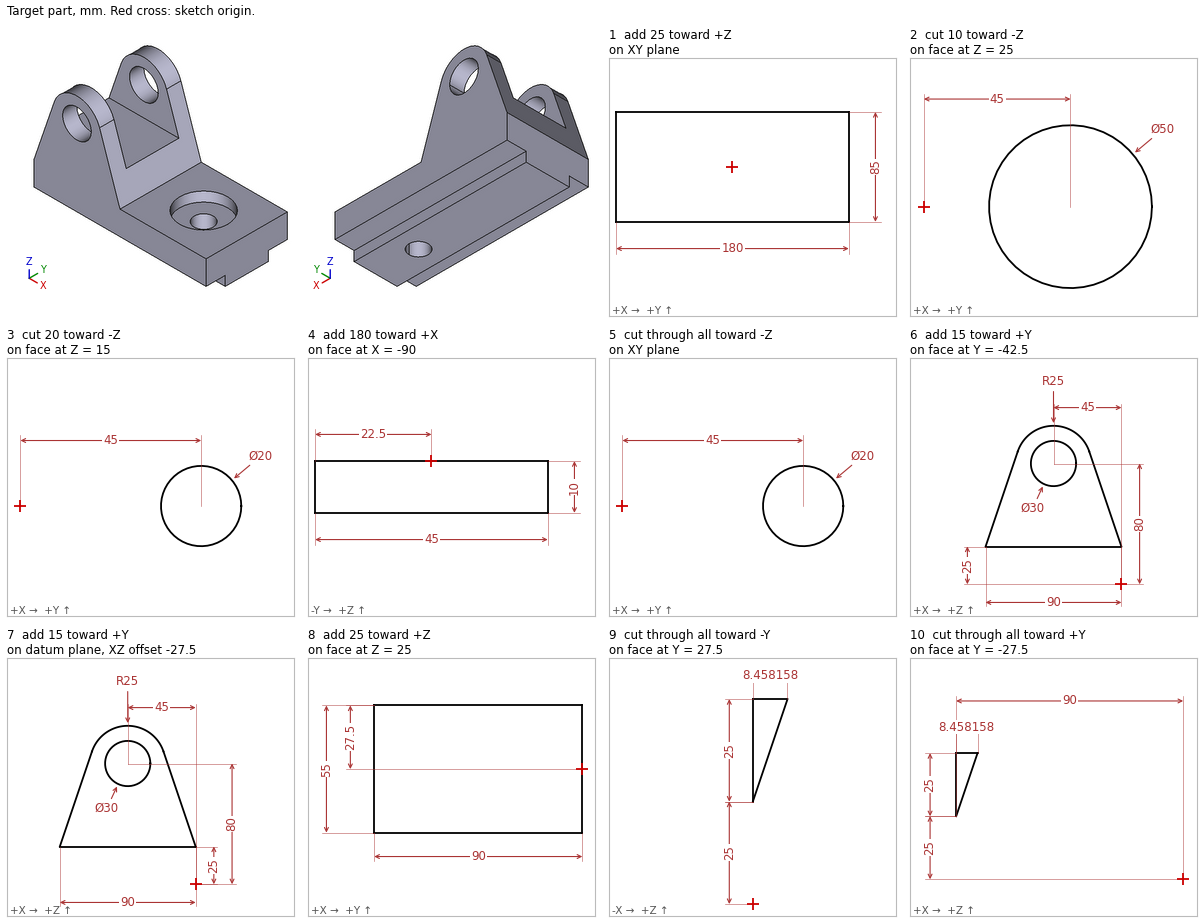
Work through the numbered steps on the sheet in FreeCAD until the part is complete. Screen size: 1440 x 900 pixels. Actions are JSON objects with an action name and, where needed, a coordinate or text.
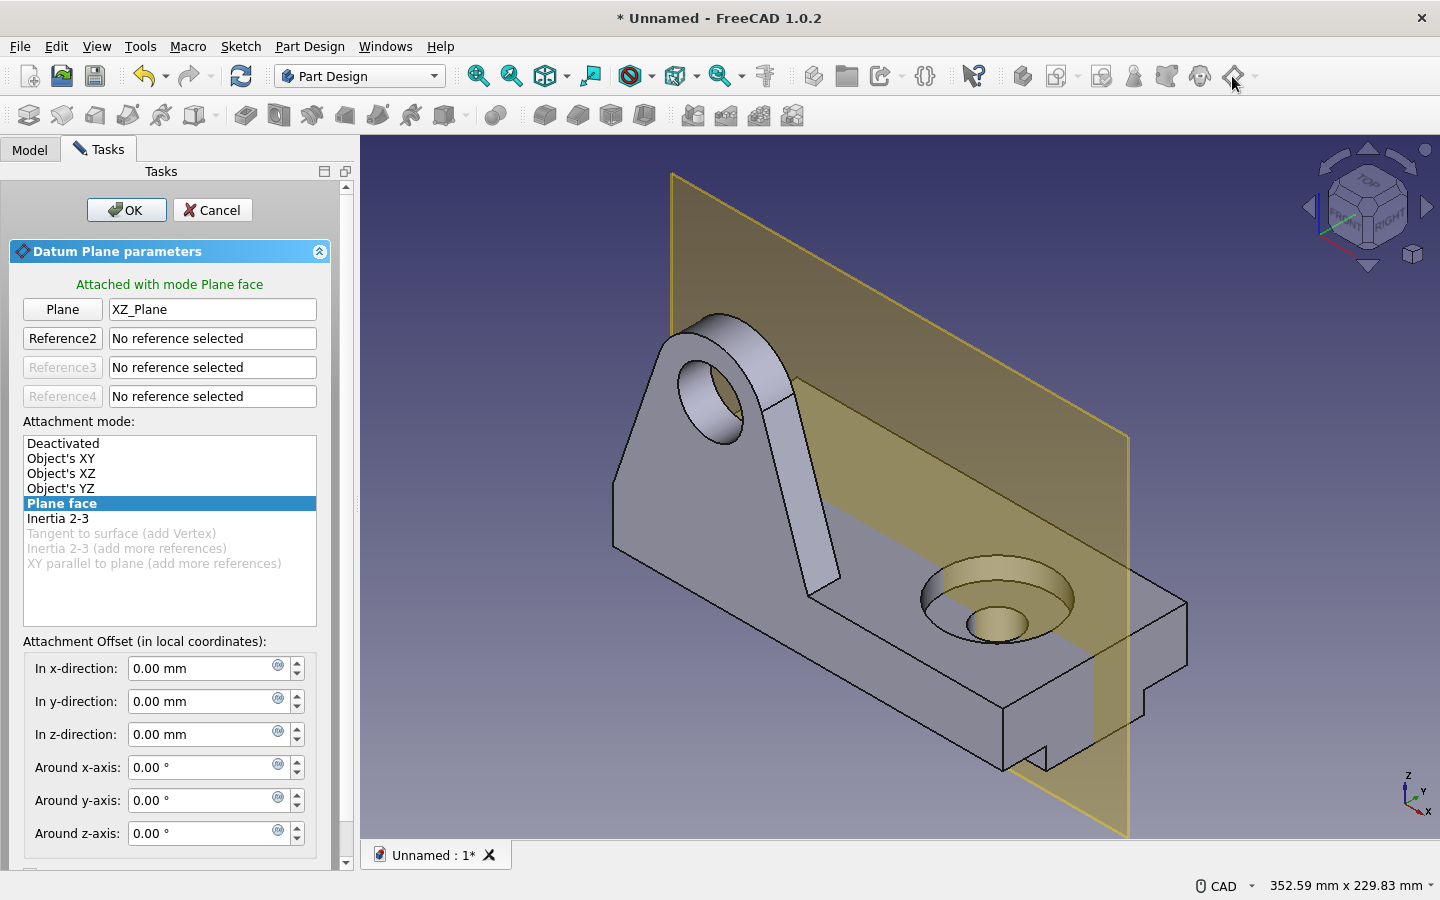
{"action": "triple_click", "coordinate": [210, 734]}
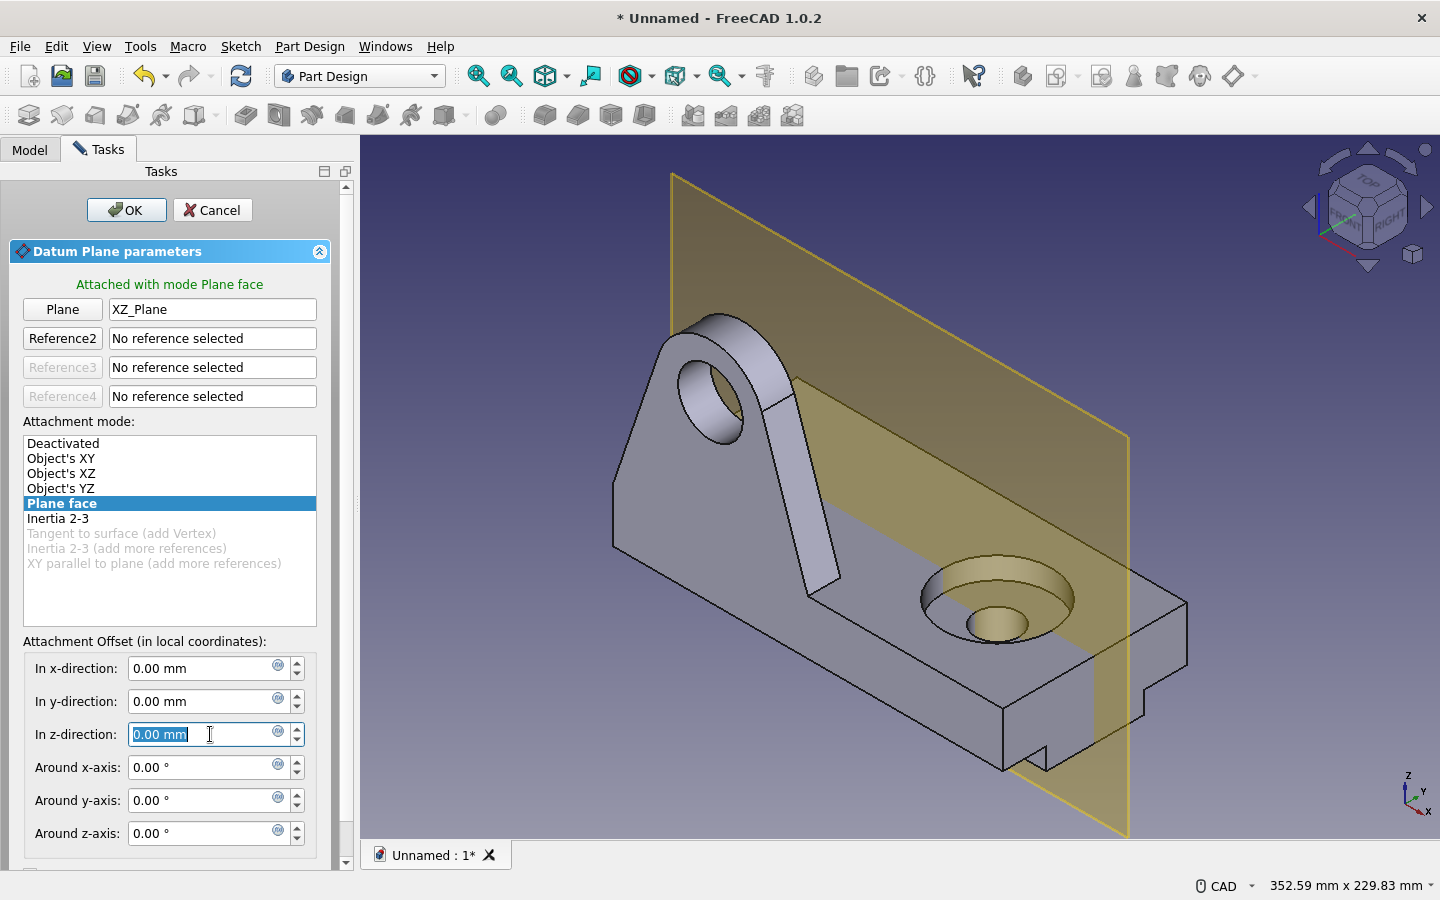
{"action": "type", "text": "-27.5"}
{"action": "key", "text": "Tab"}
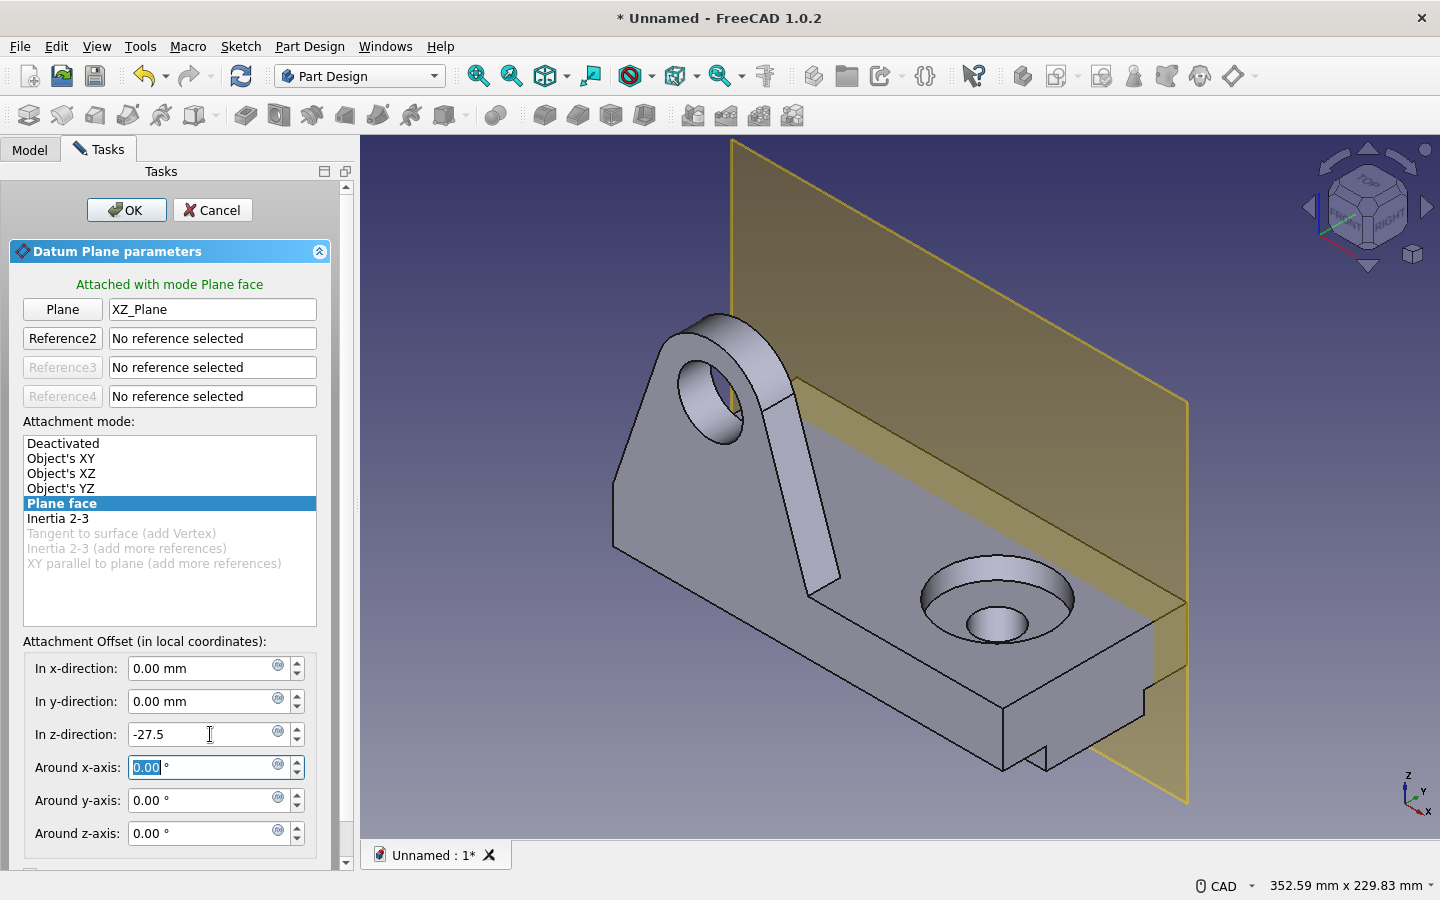
{"action": "left_click", "coordinate": [127, 210]}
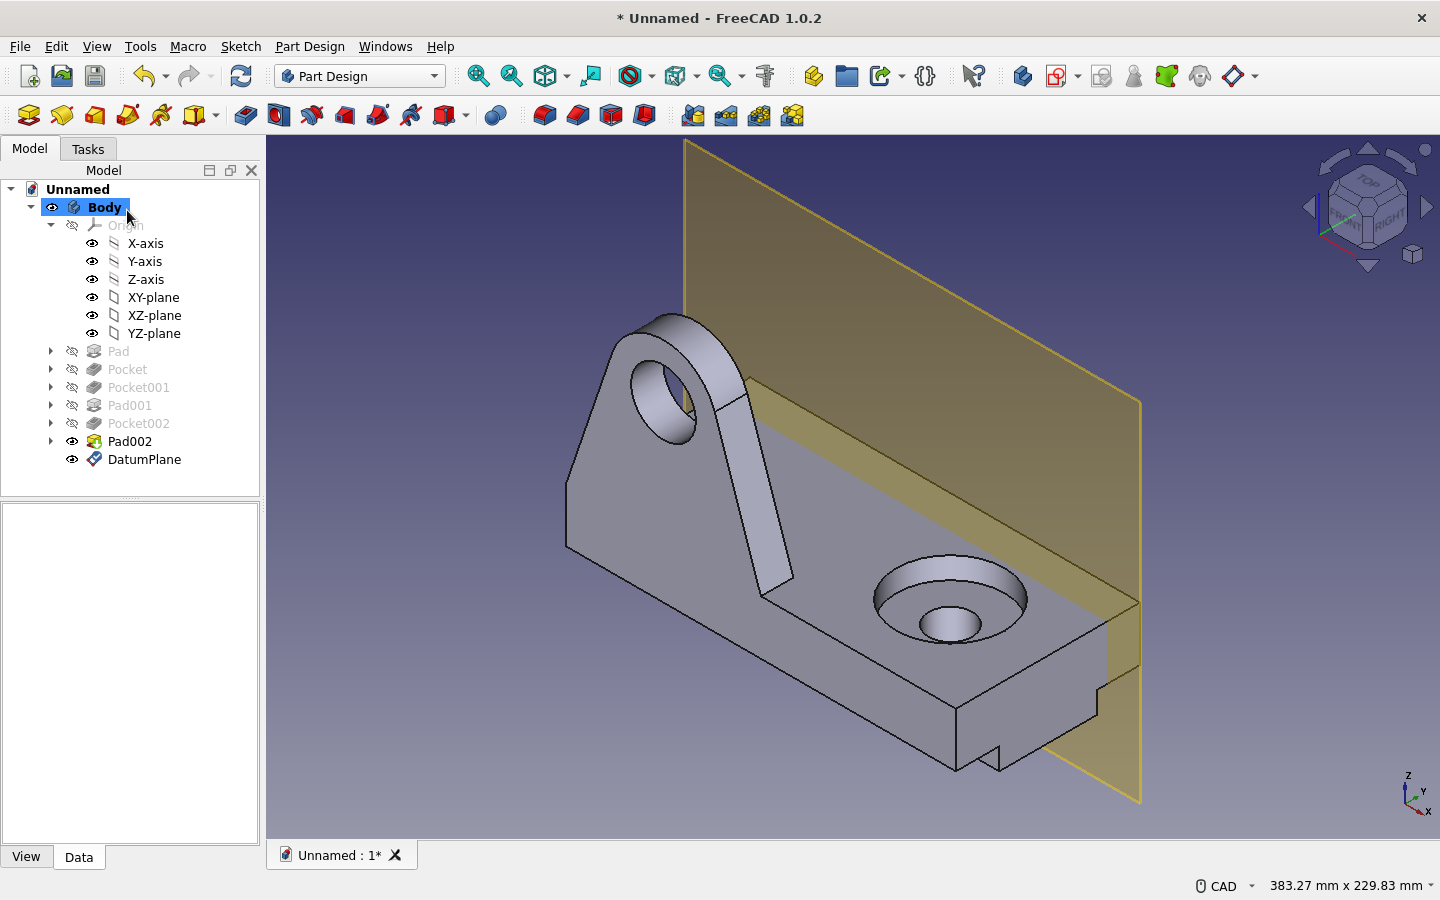
{"action": "left_click", "coordinate": [117, 459]}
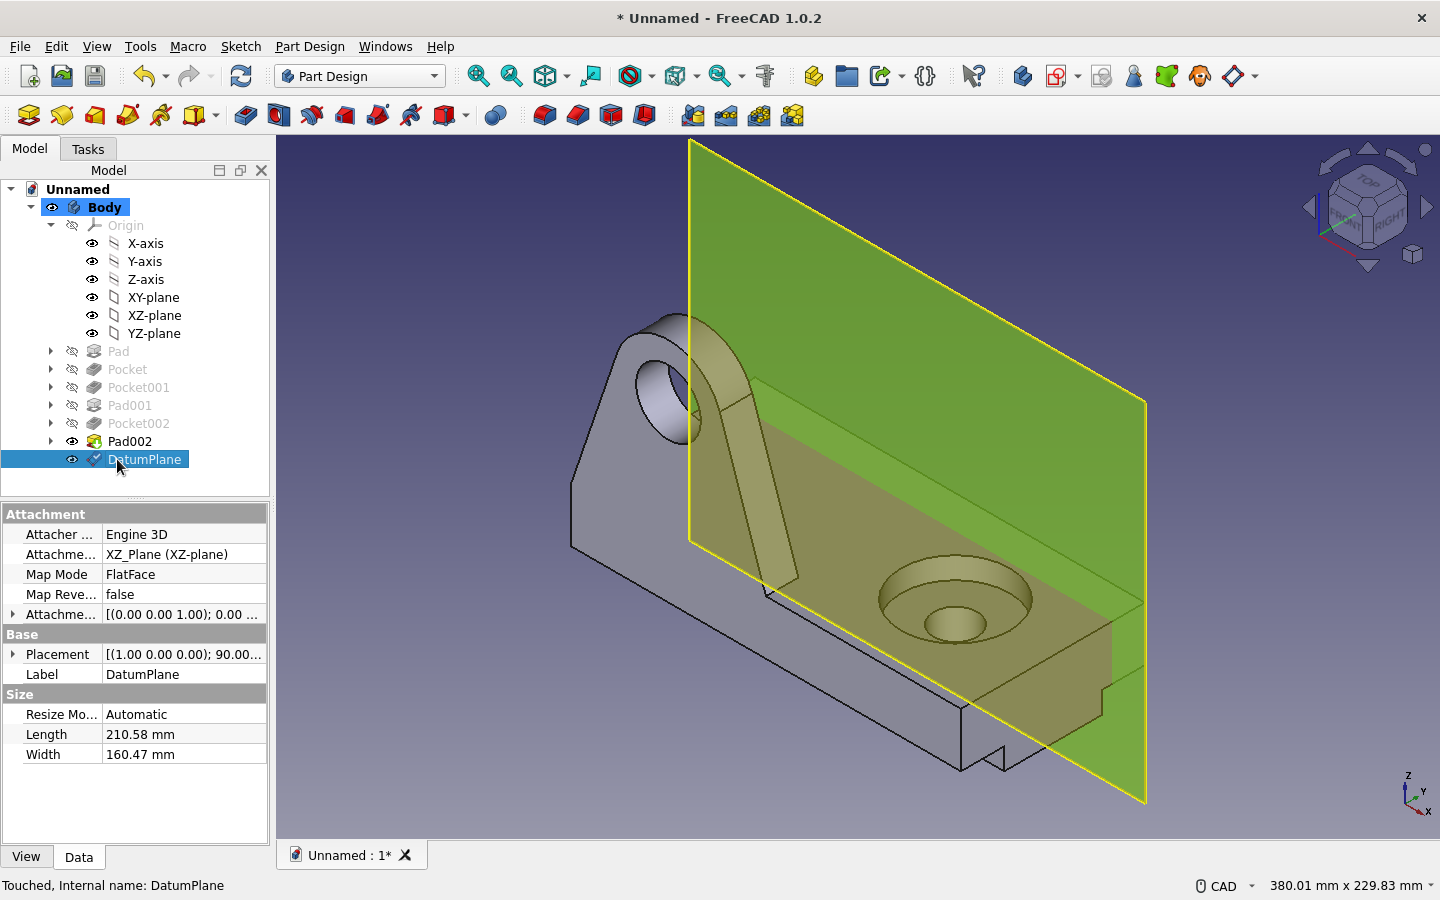
{"action": "left_click", "coordinate": [1056, 76]}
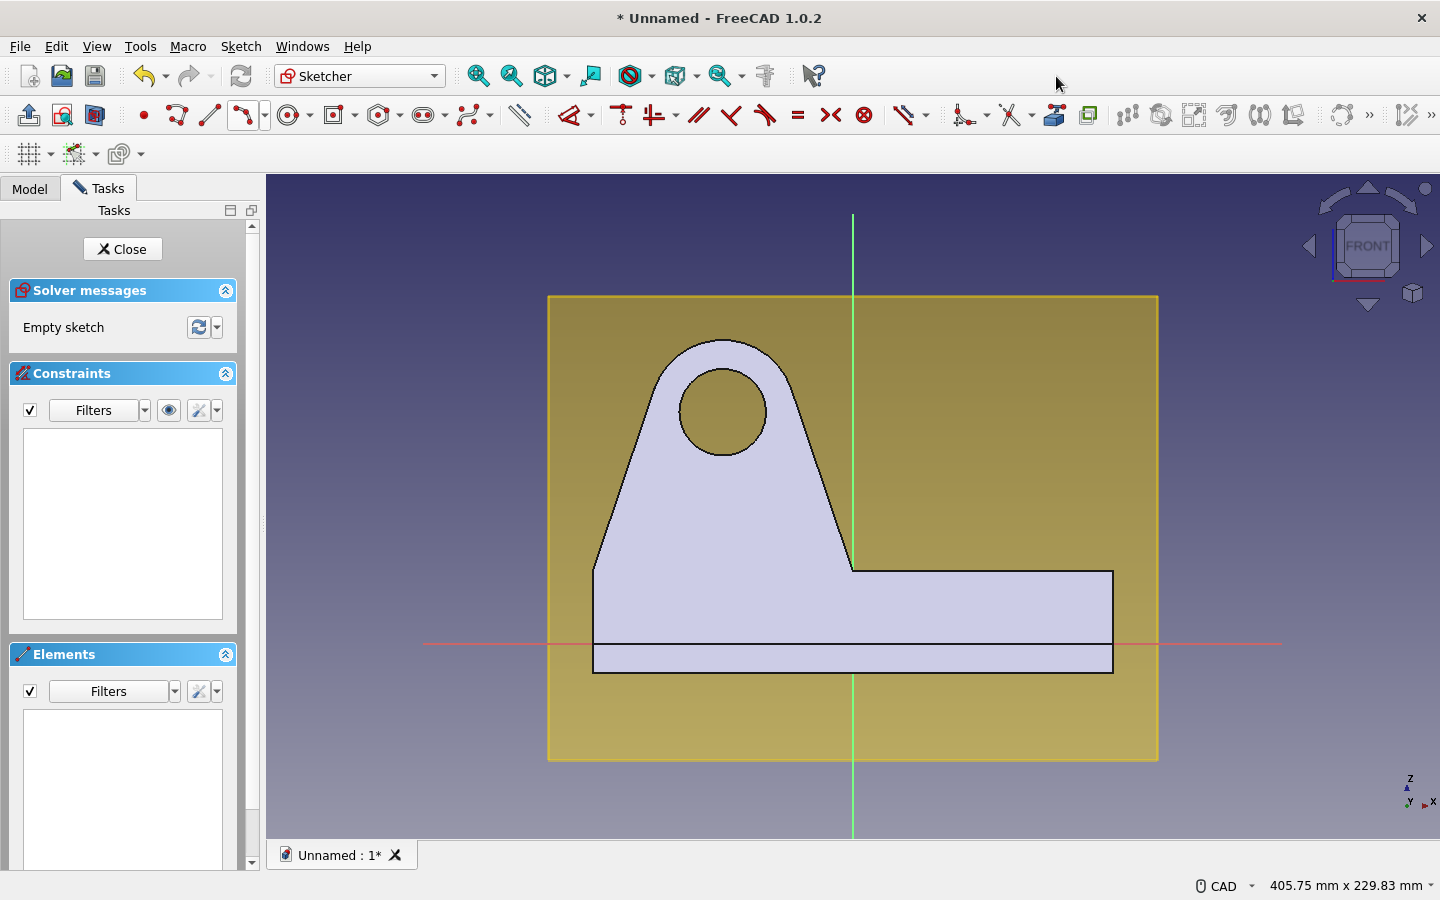
{"action": "left_click", "coordinate": [95, 116]}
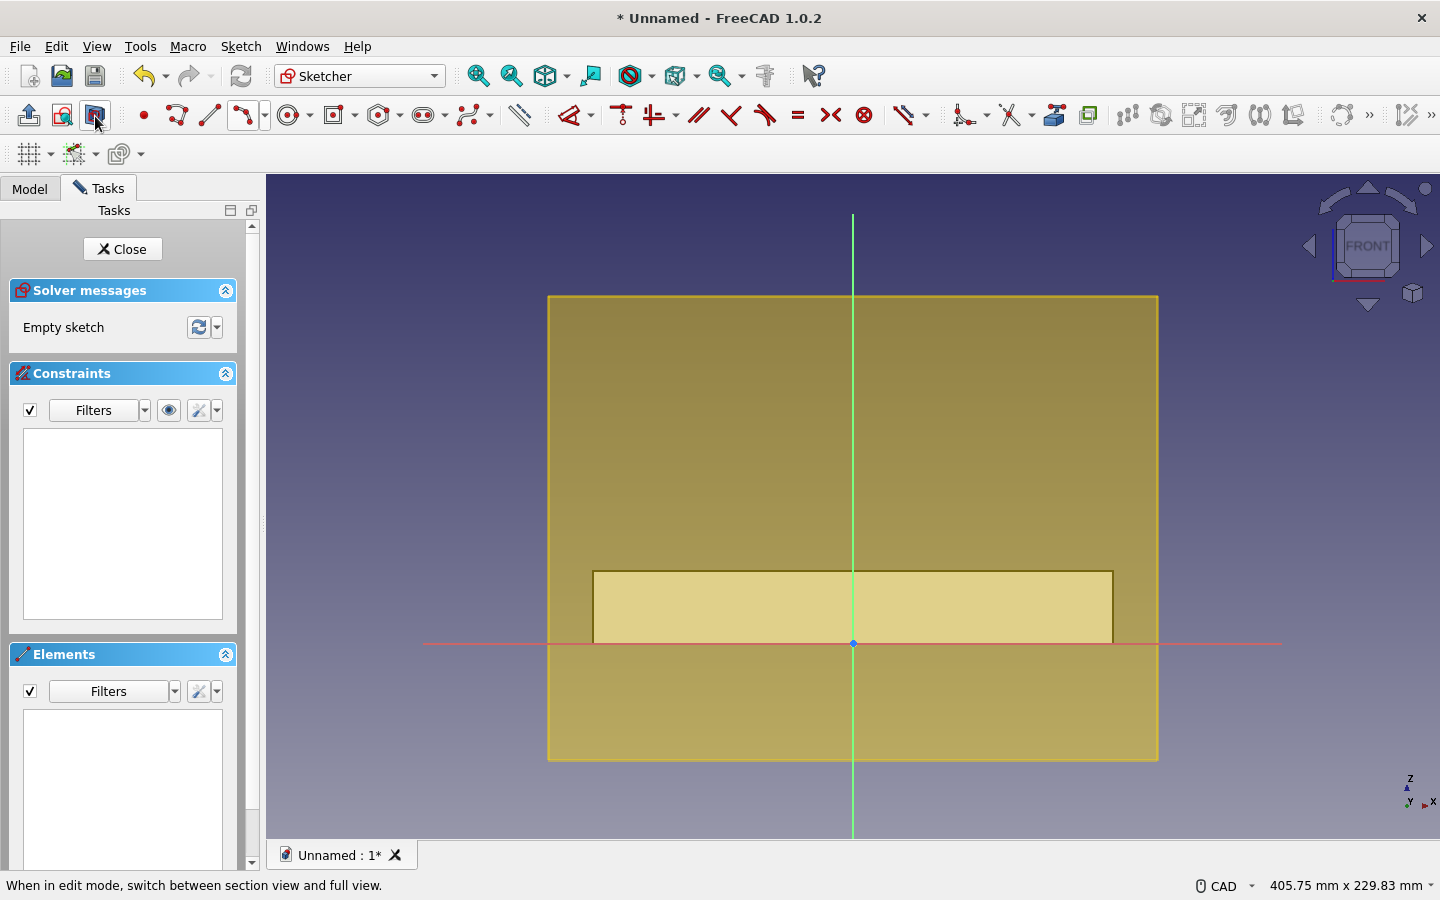
{"action": "scroll", "coordinate": [597, 462], "scroll_direction": "up", "scroll_amount": 2}